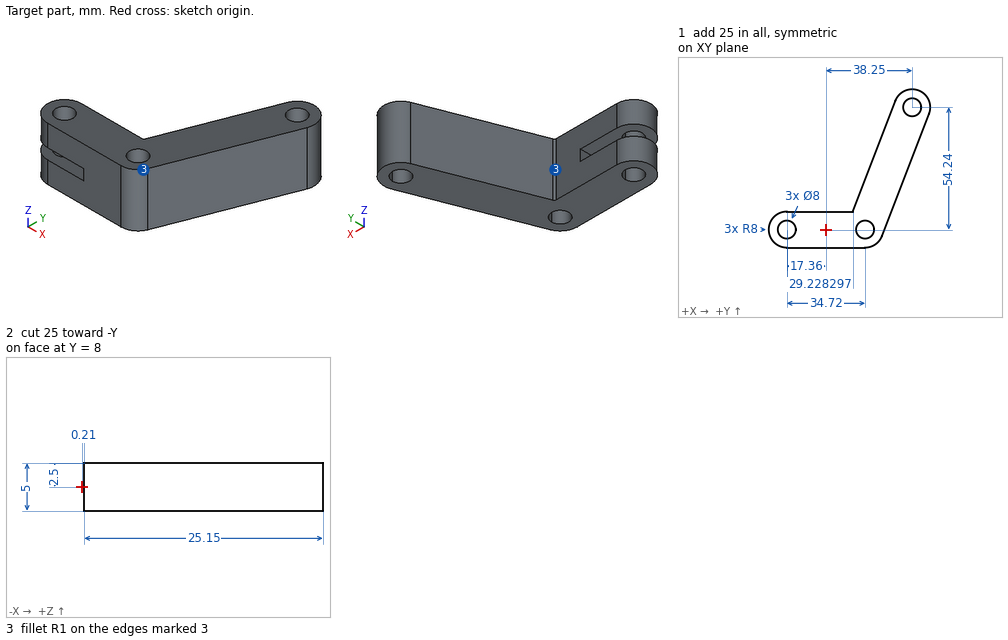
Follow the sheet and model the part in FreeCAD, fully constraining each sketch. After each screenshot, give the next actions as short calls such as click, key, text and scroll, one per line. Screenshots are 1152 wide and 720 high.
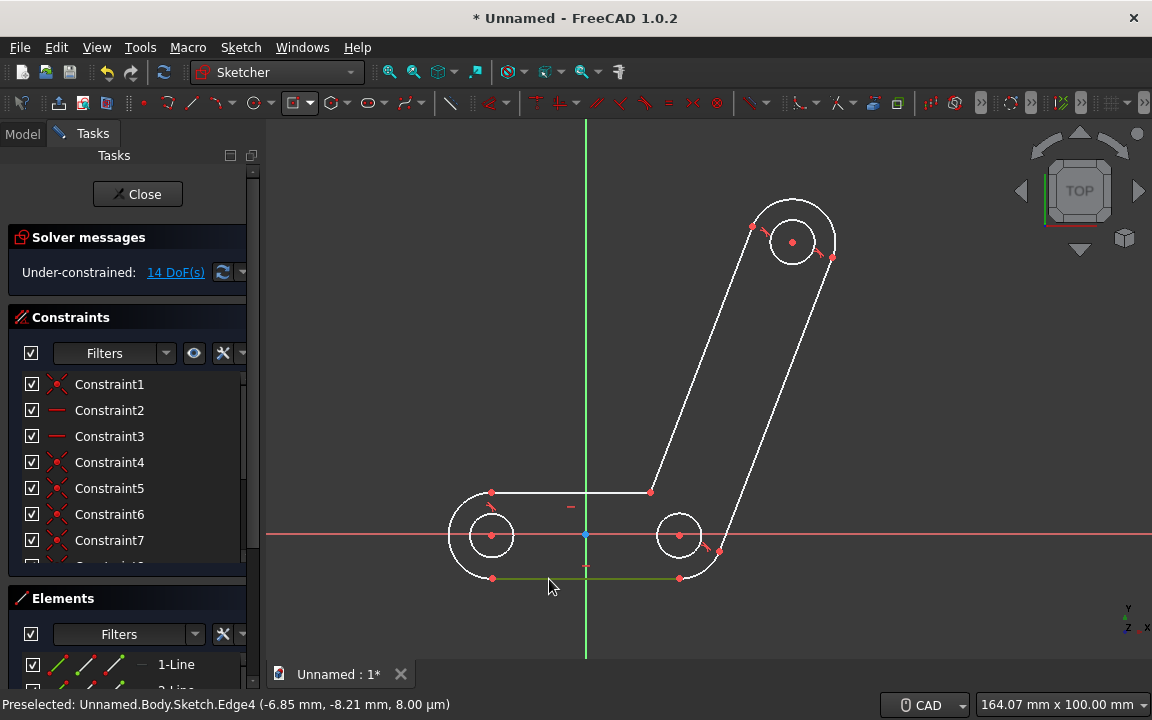
click(457, 510)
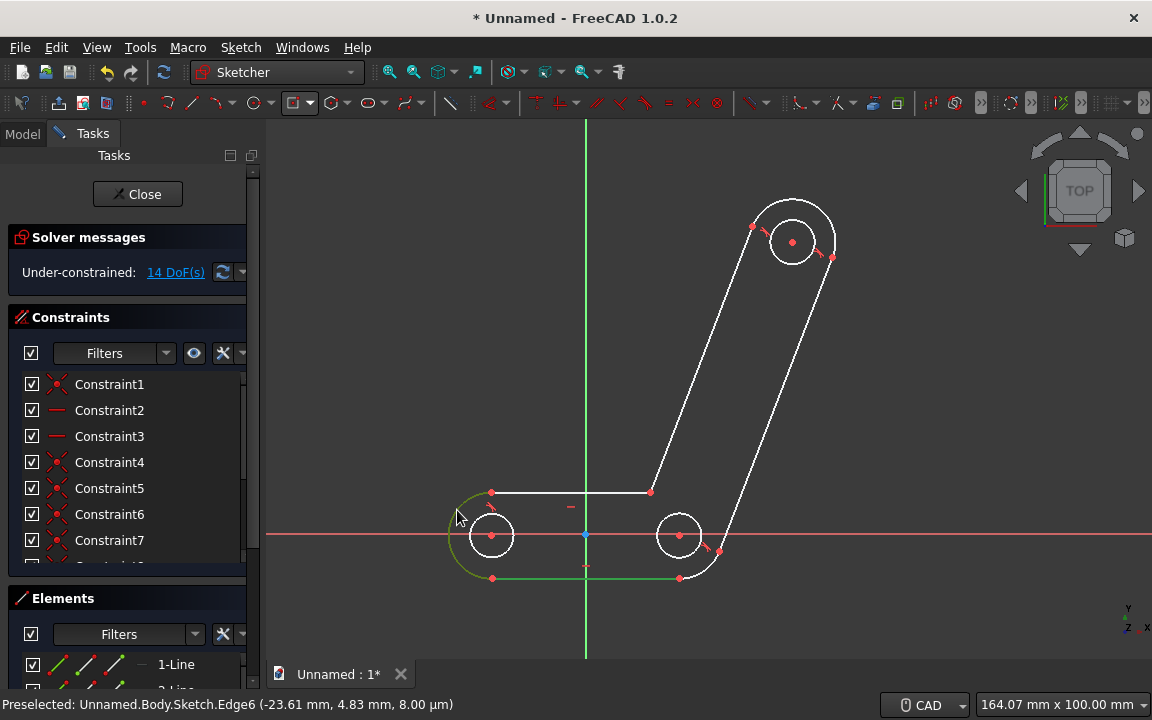
key(t)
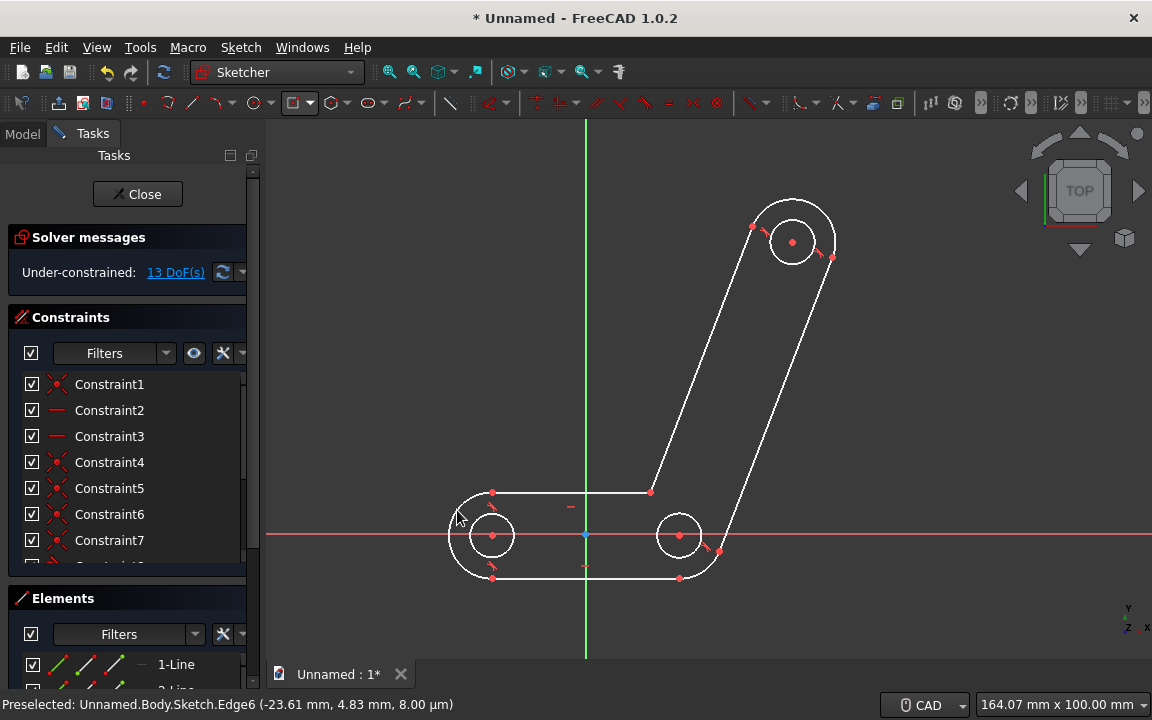
click(548, 579)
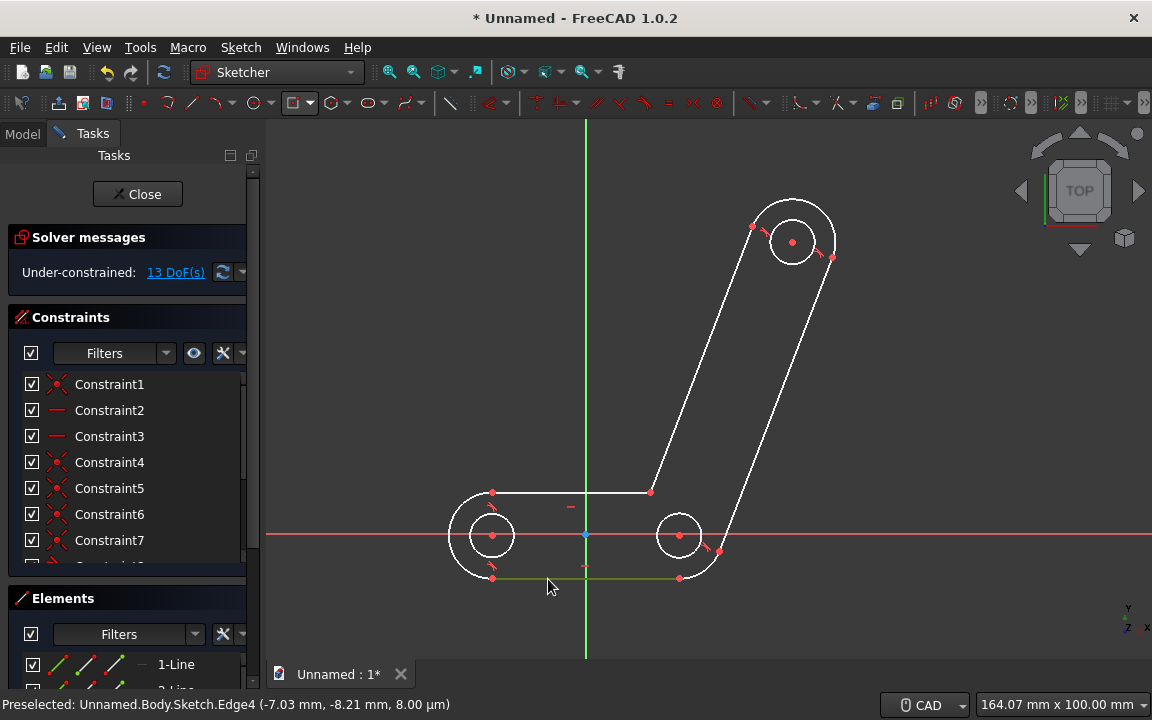
click(695, 576)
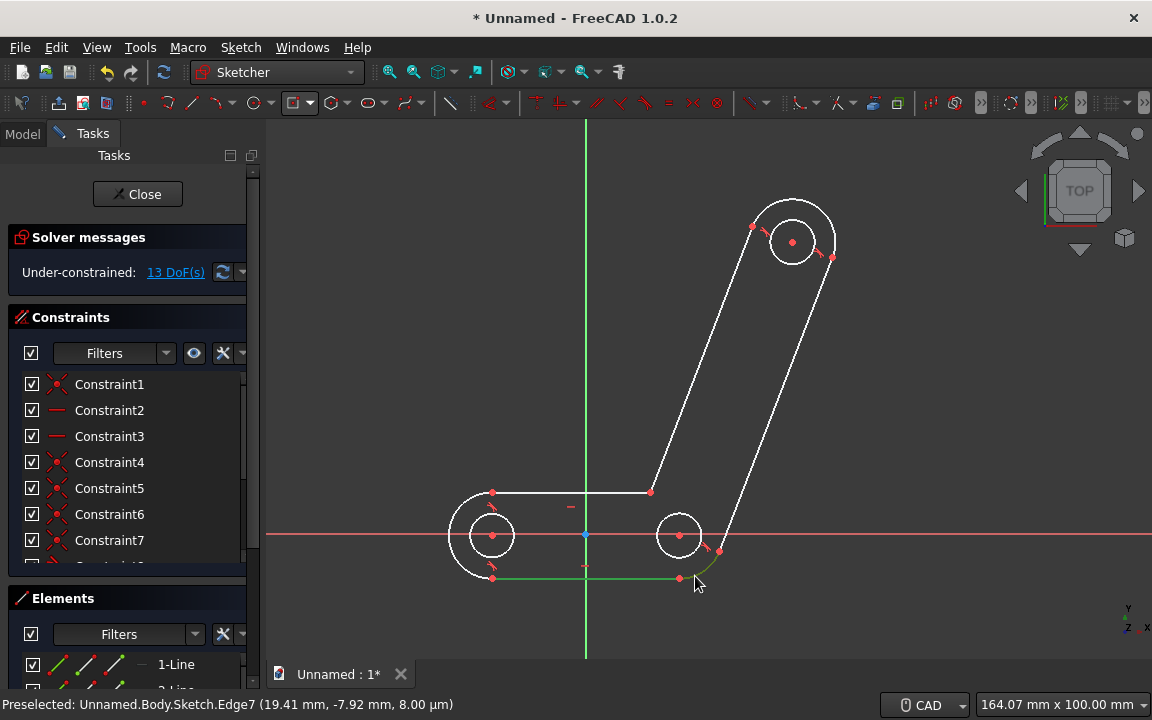
click(646, 104)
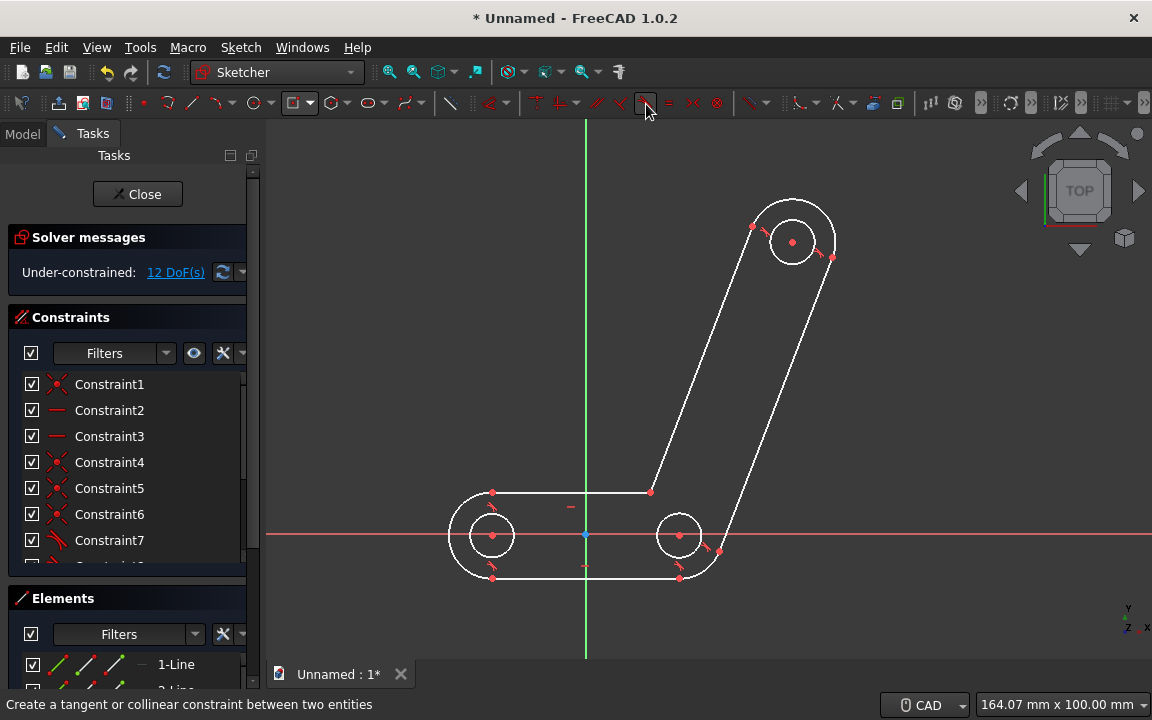
click(829, 219)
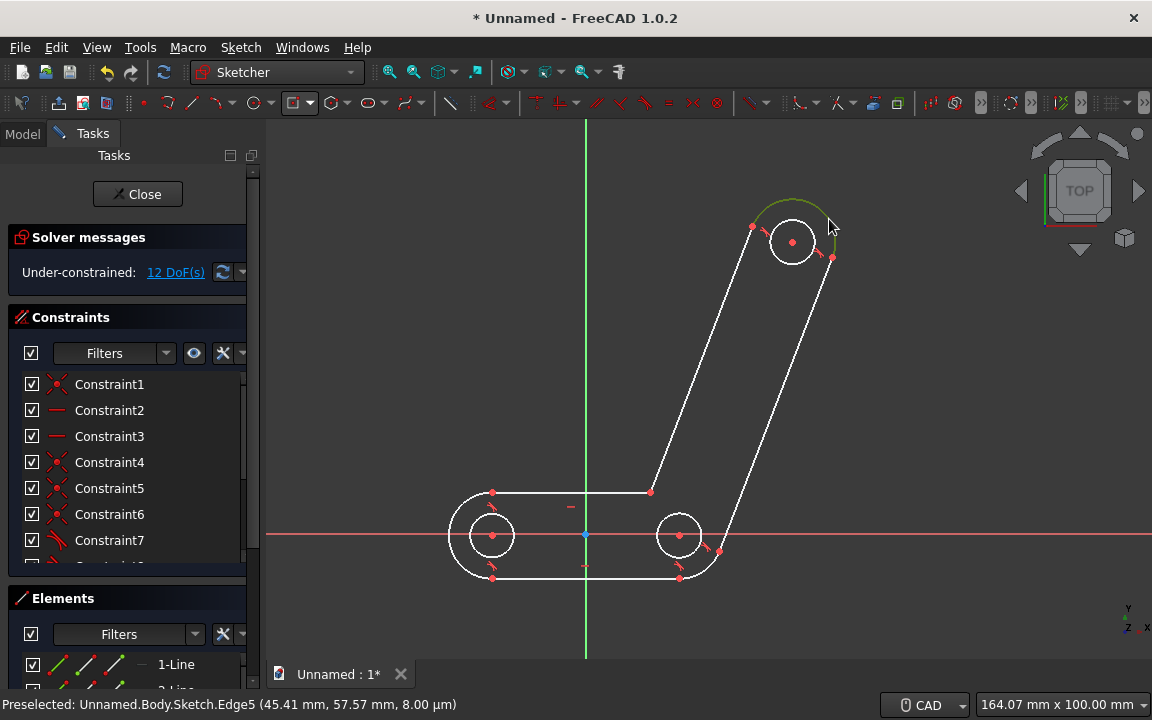
click(457, 510)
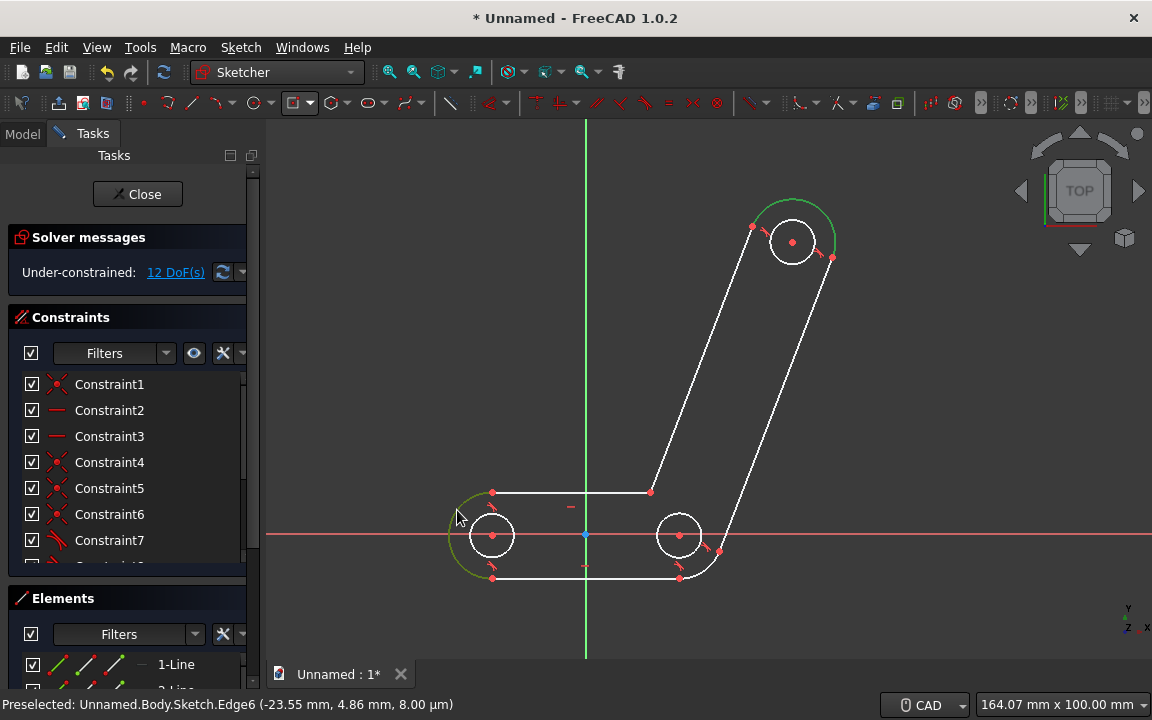
click(695, 576)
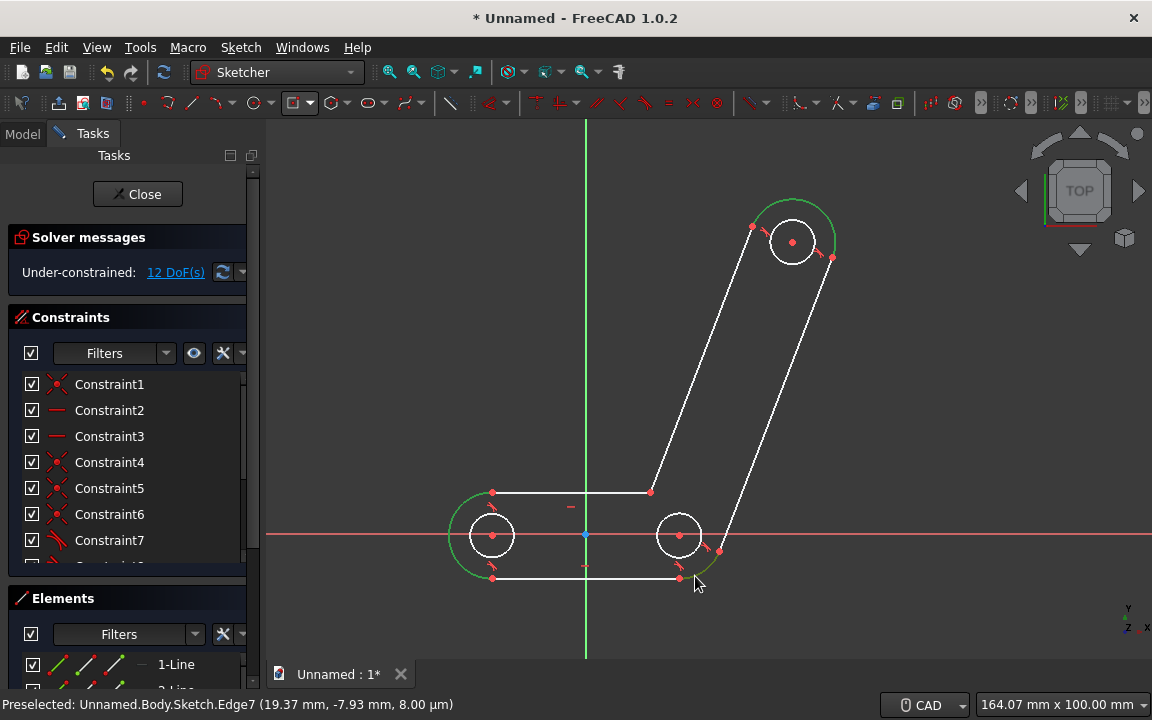
click(670, 104)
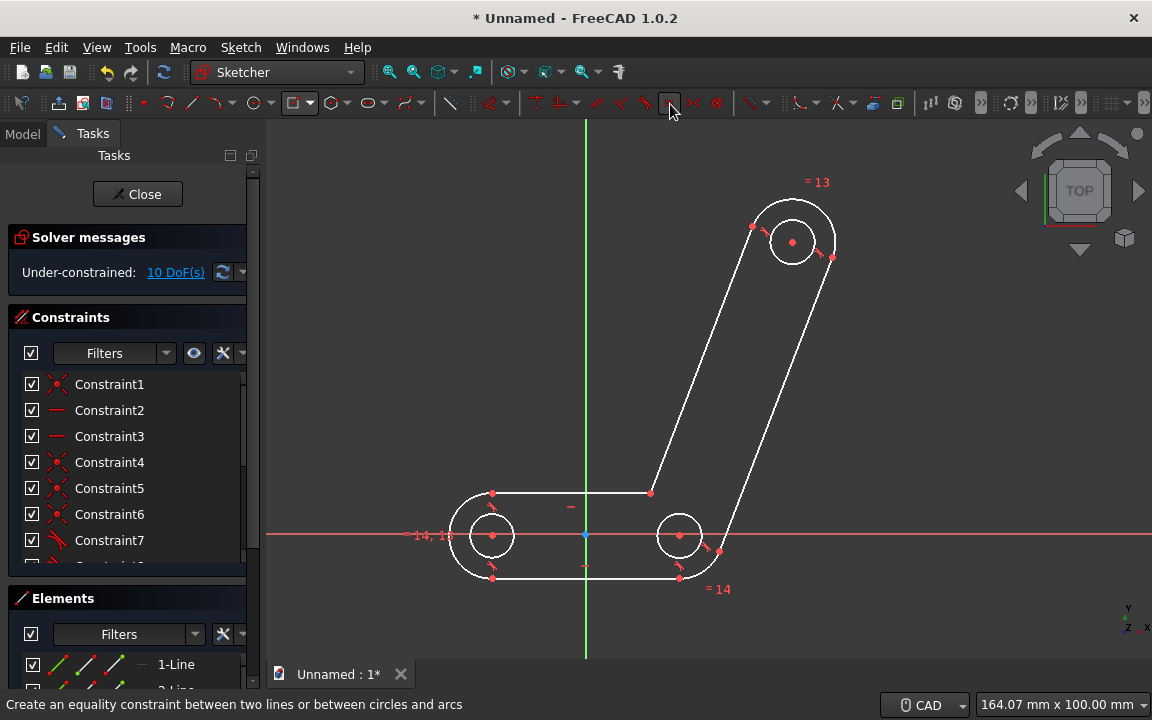
click(507, 520)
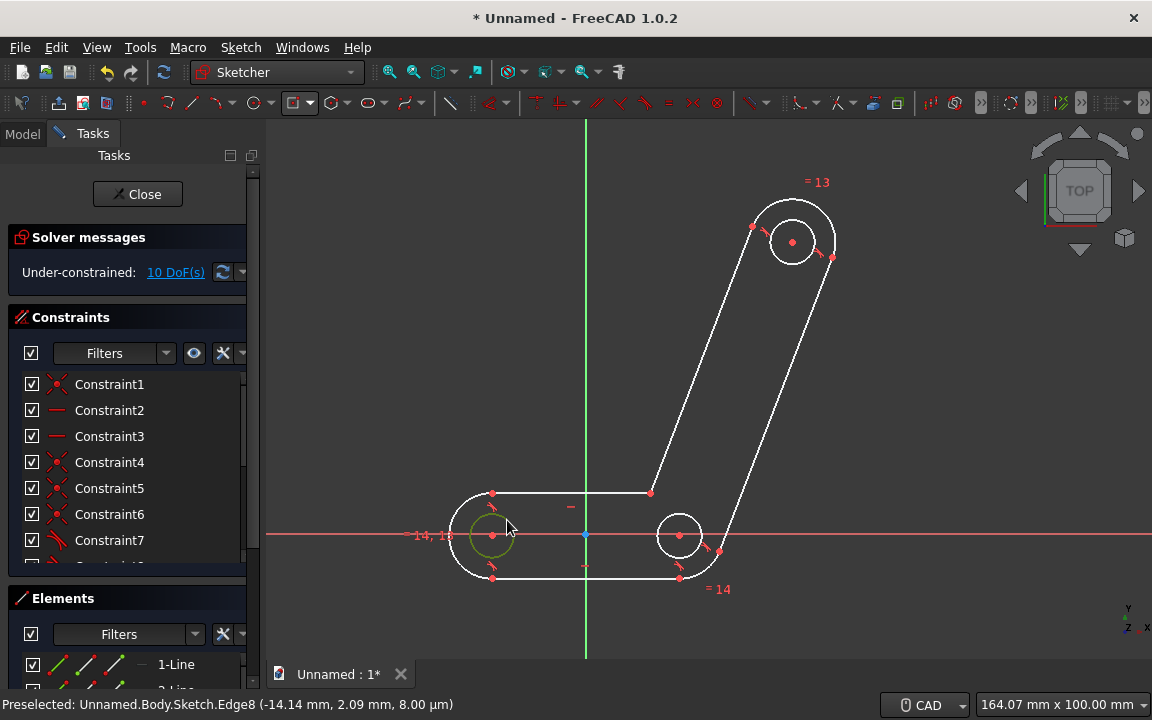
click(695, 520)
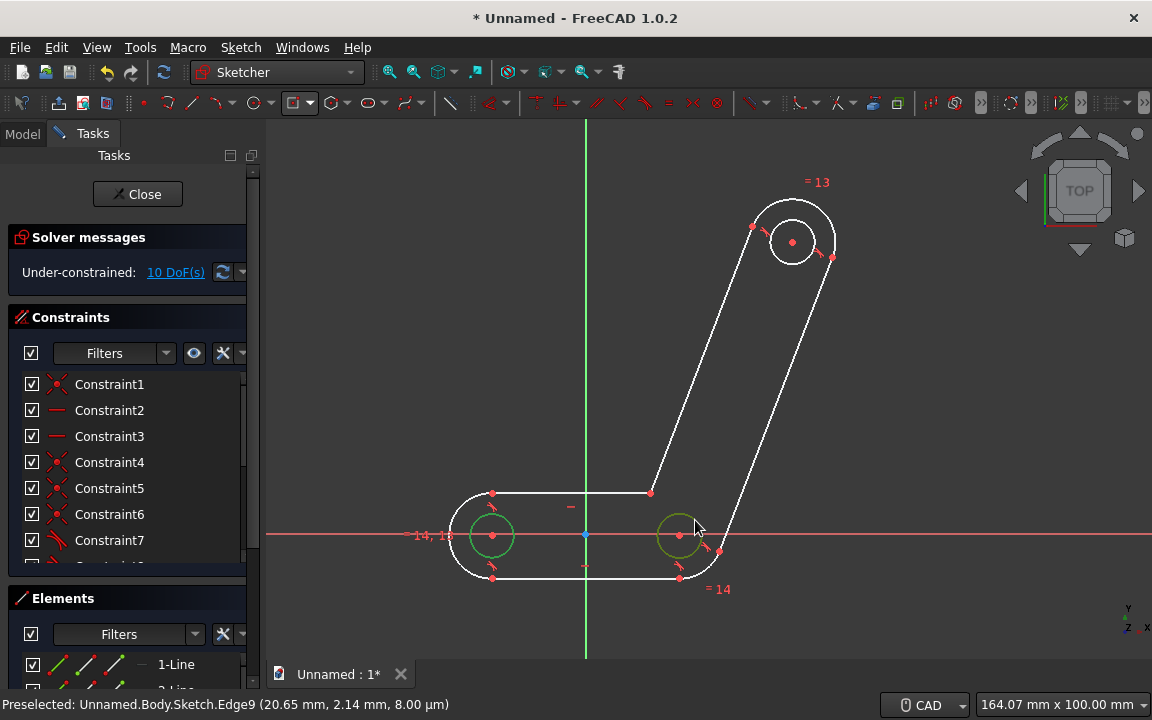
click(808, 226)